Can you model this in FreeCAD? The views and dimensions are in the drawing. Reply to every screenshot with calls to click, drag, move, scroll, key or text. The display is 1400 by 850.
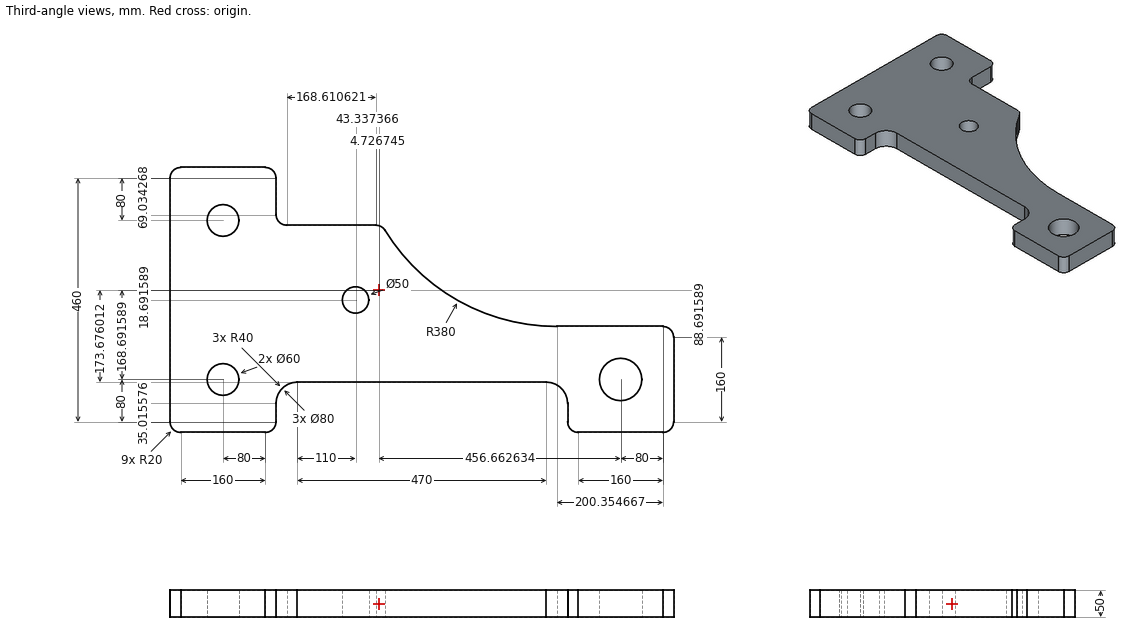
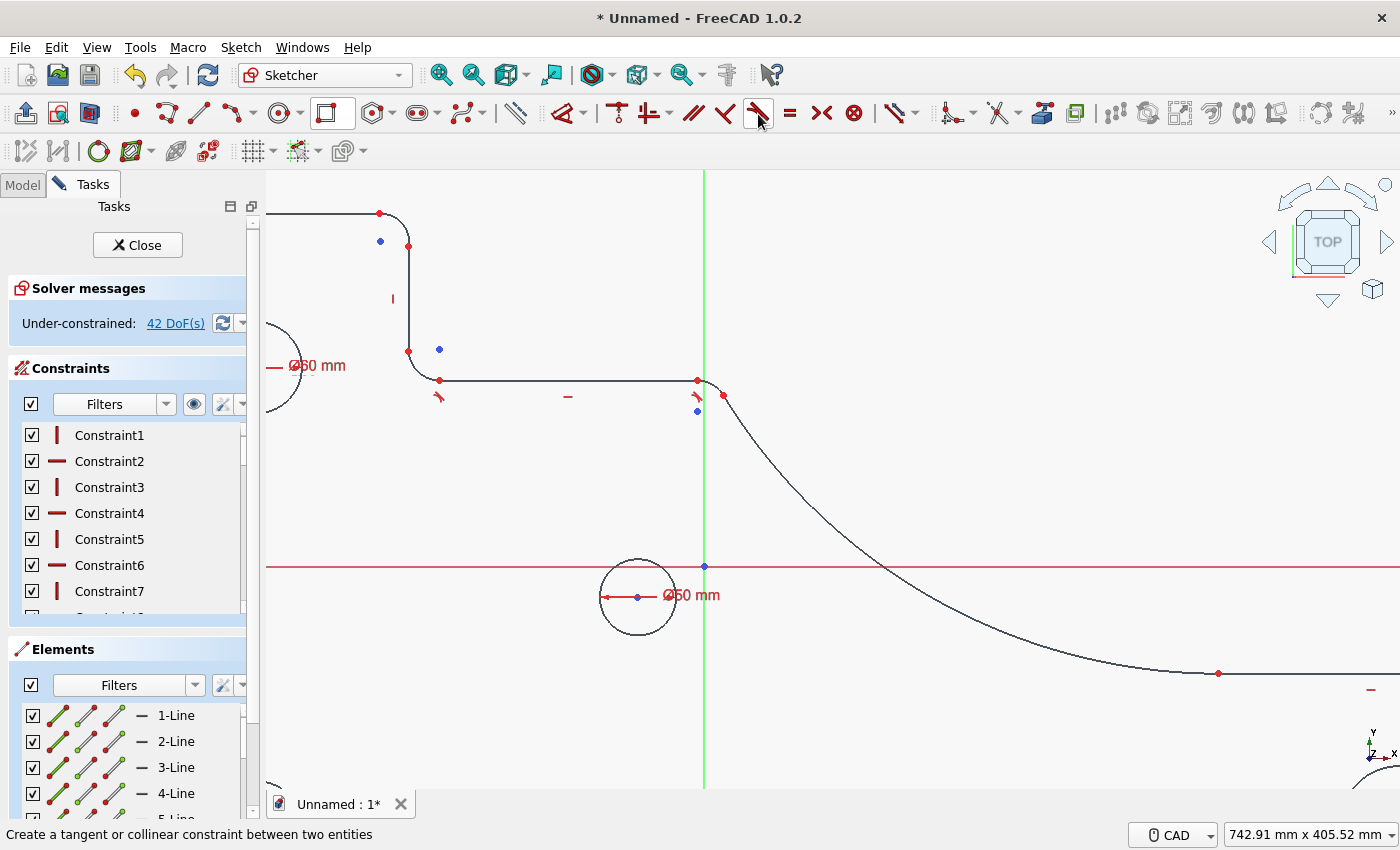
click(409, 320)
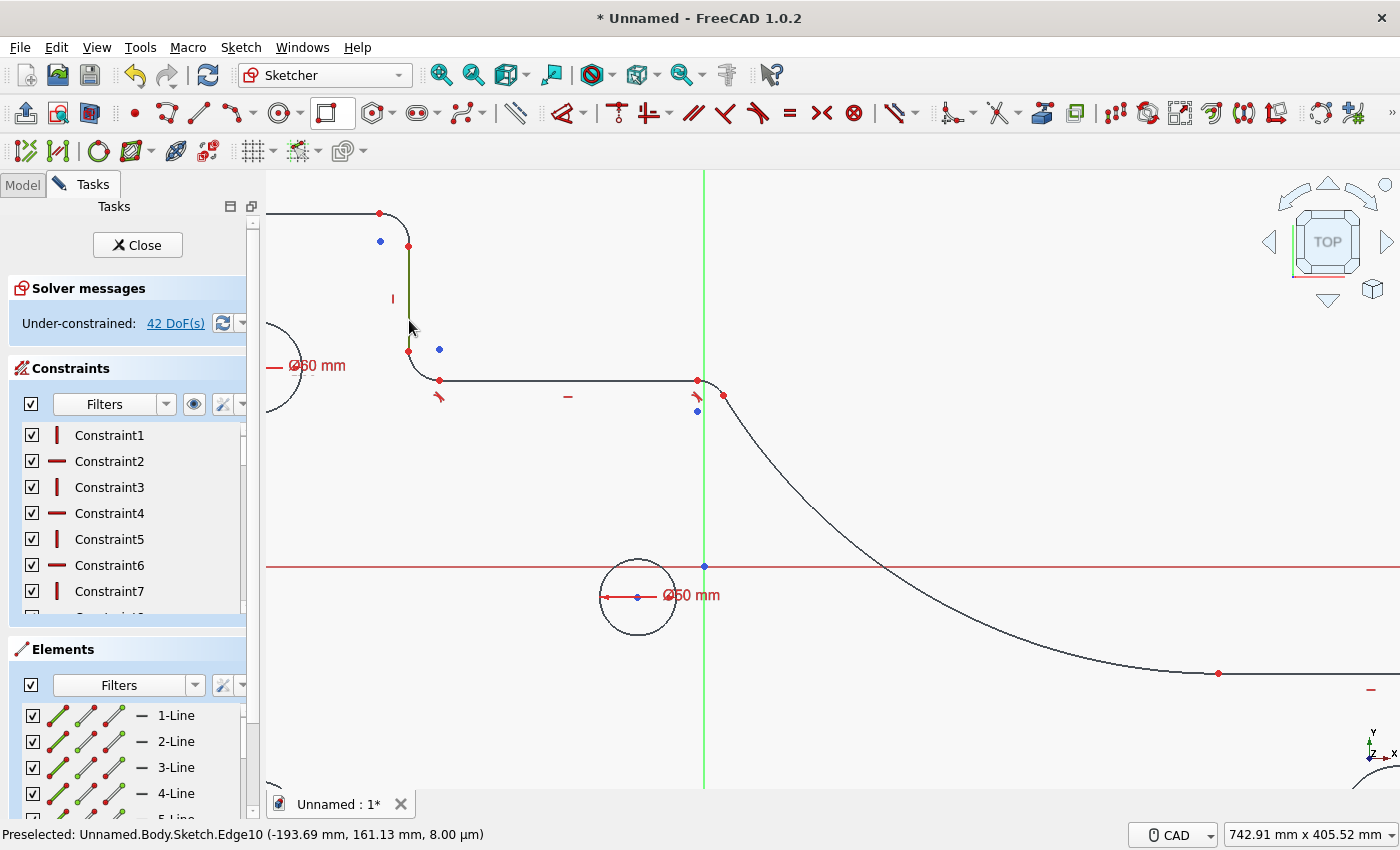
click(413, 365)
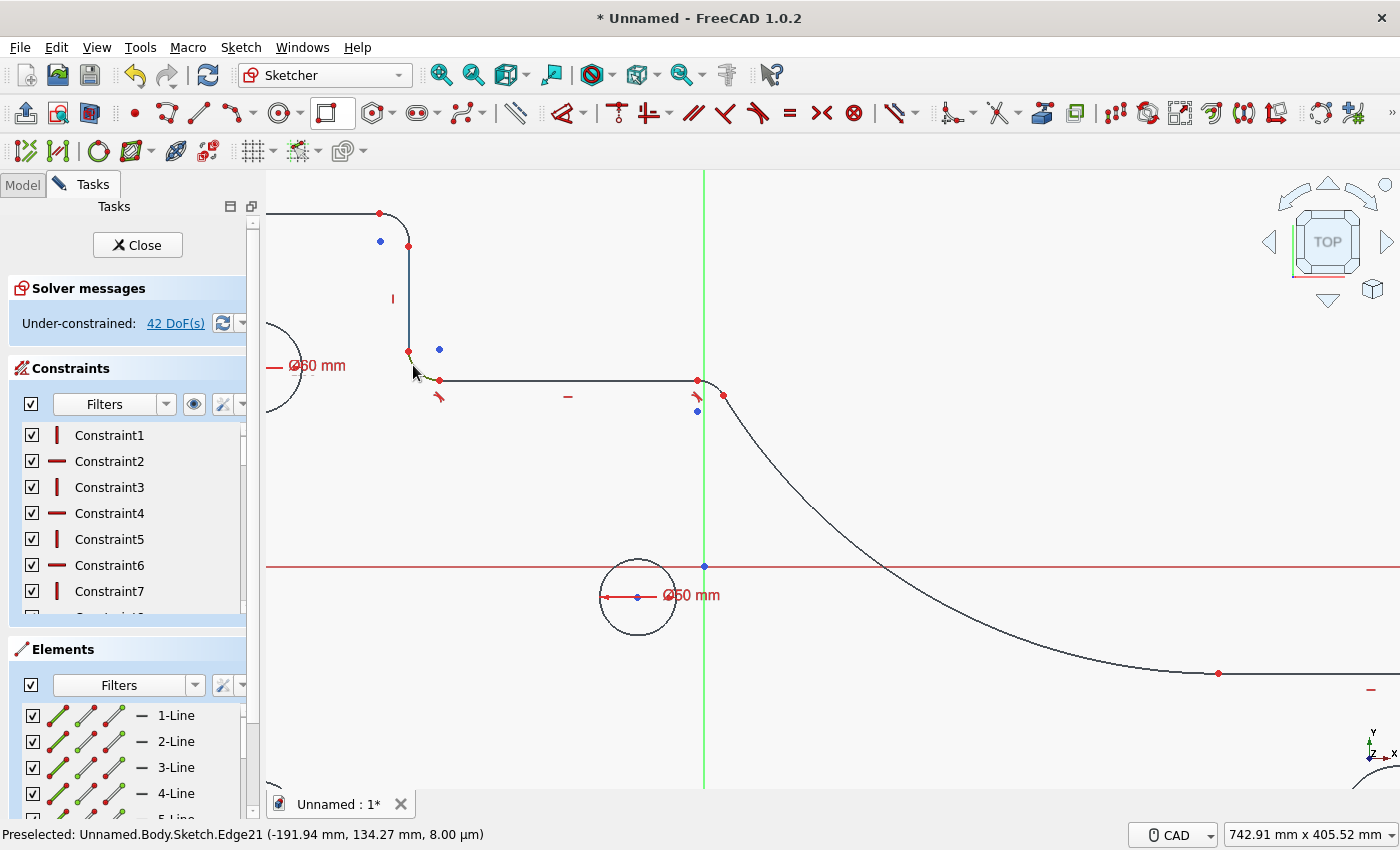
click(758, 114)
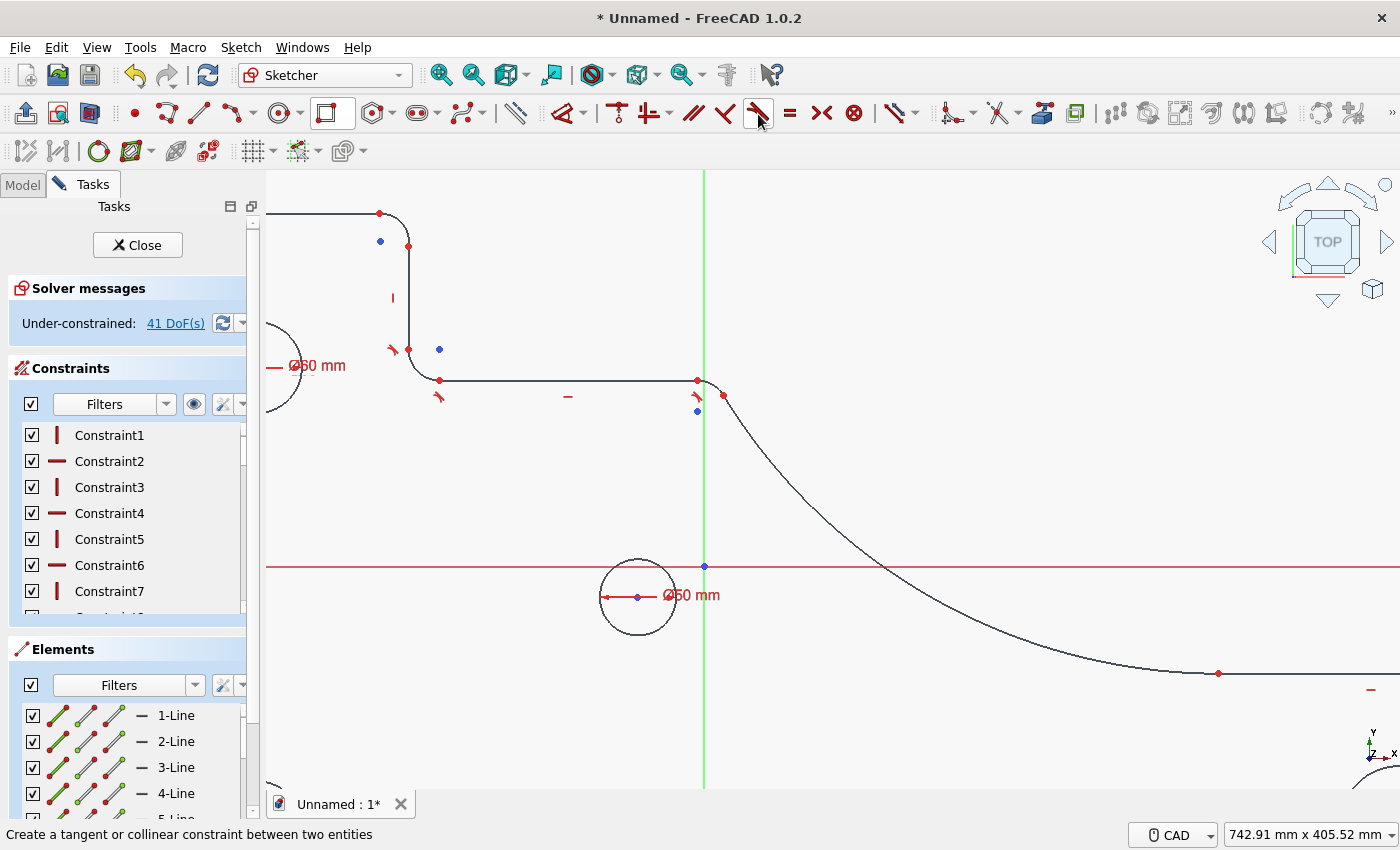
click(409, 318)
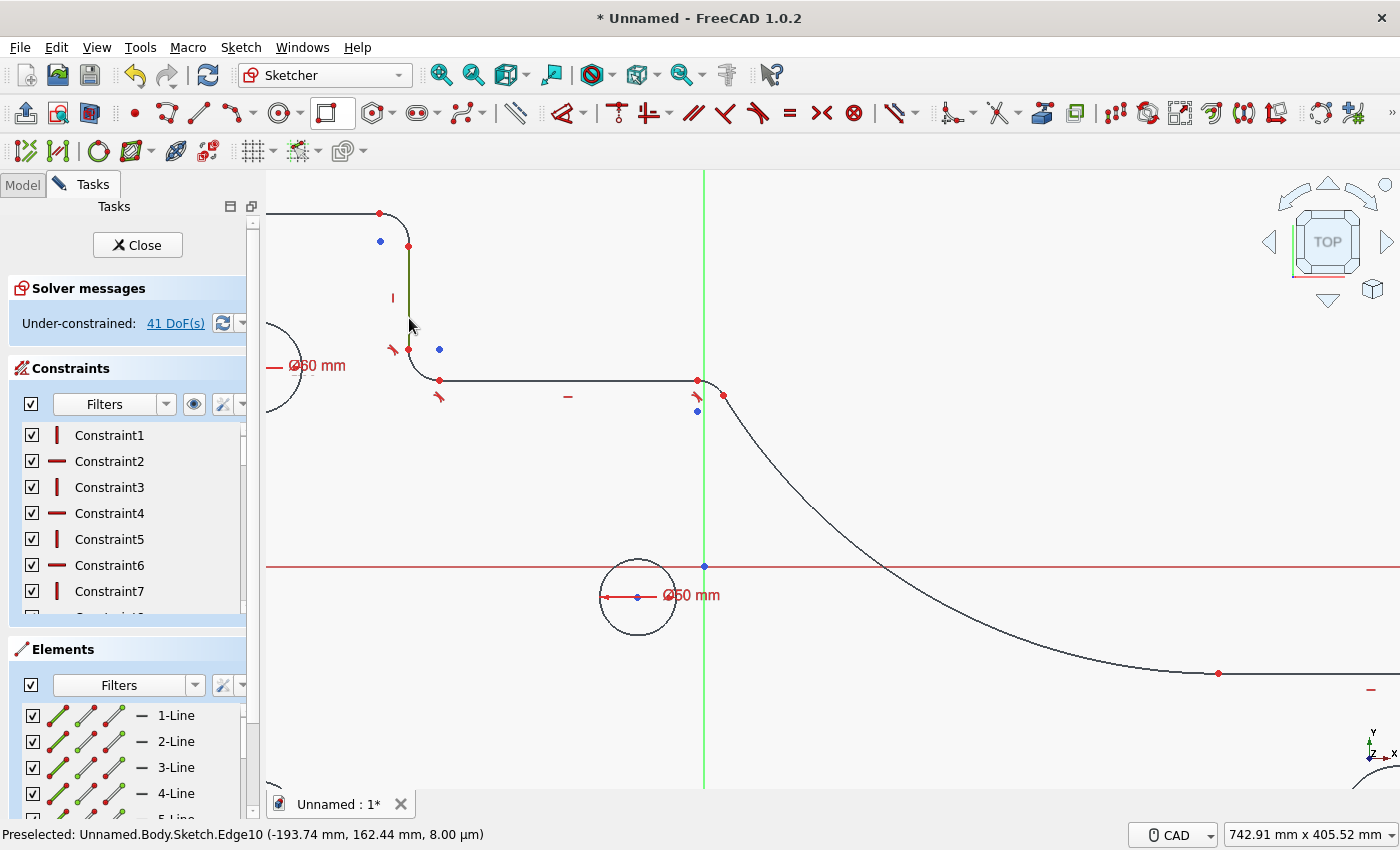
click(407, 232)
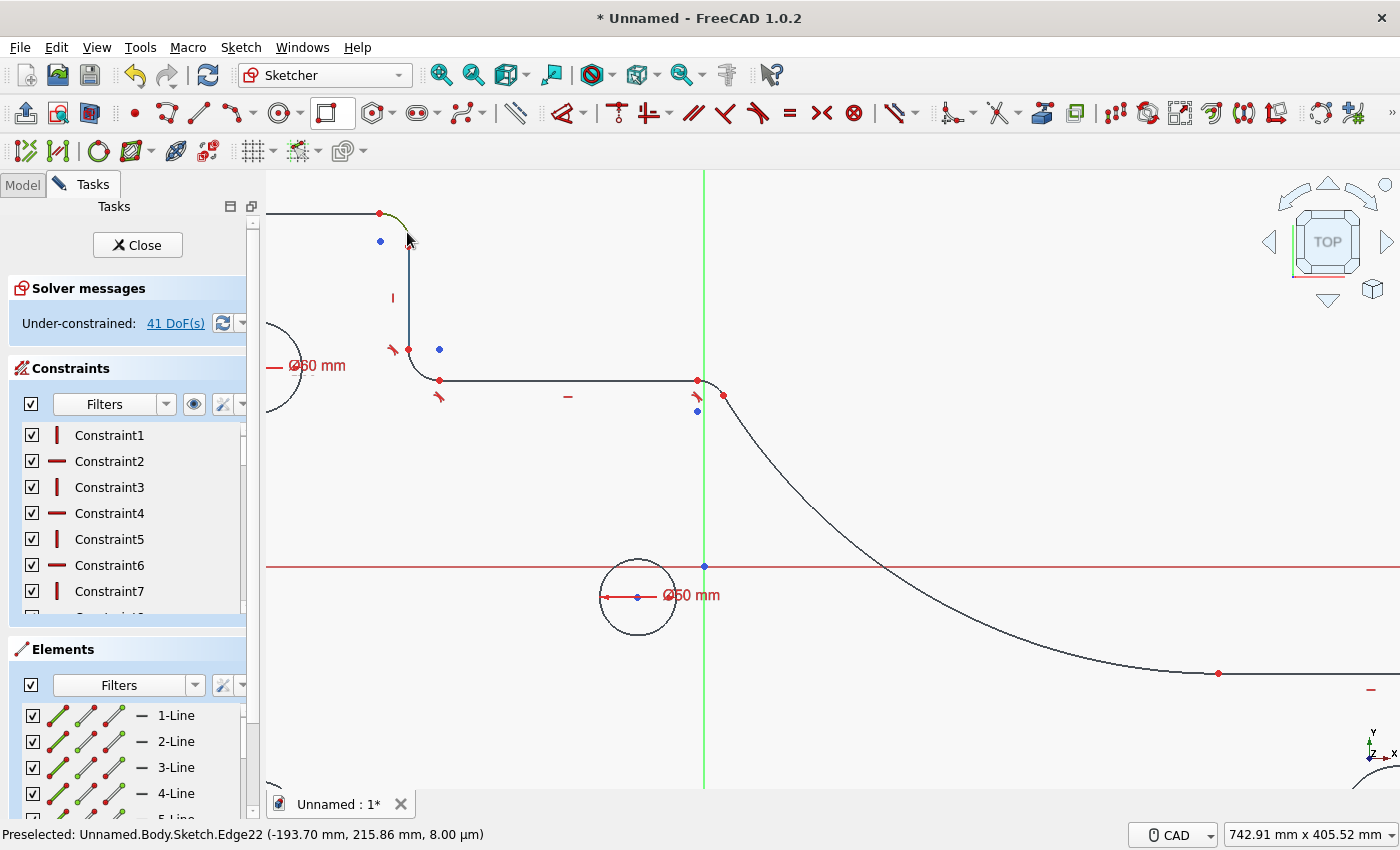
click(758, 114)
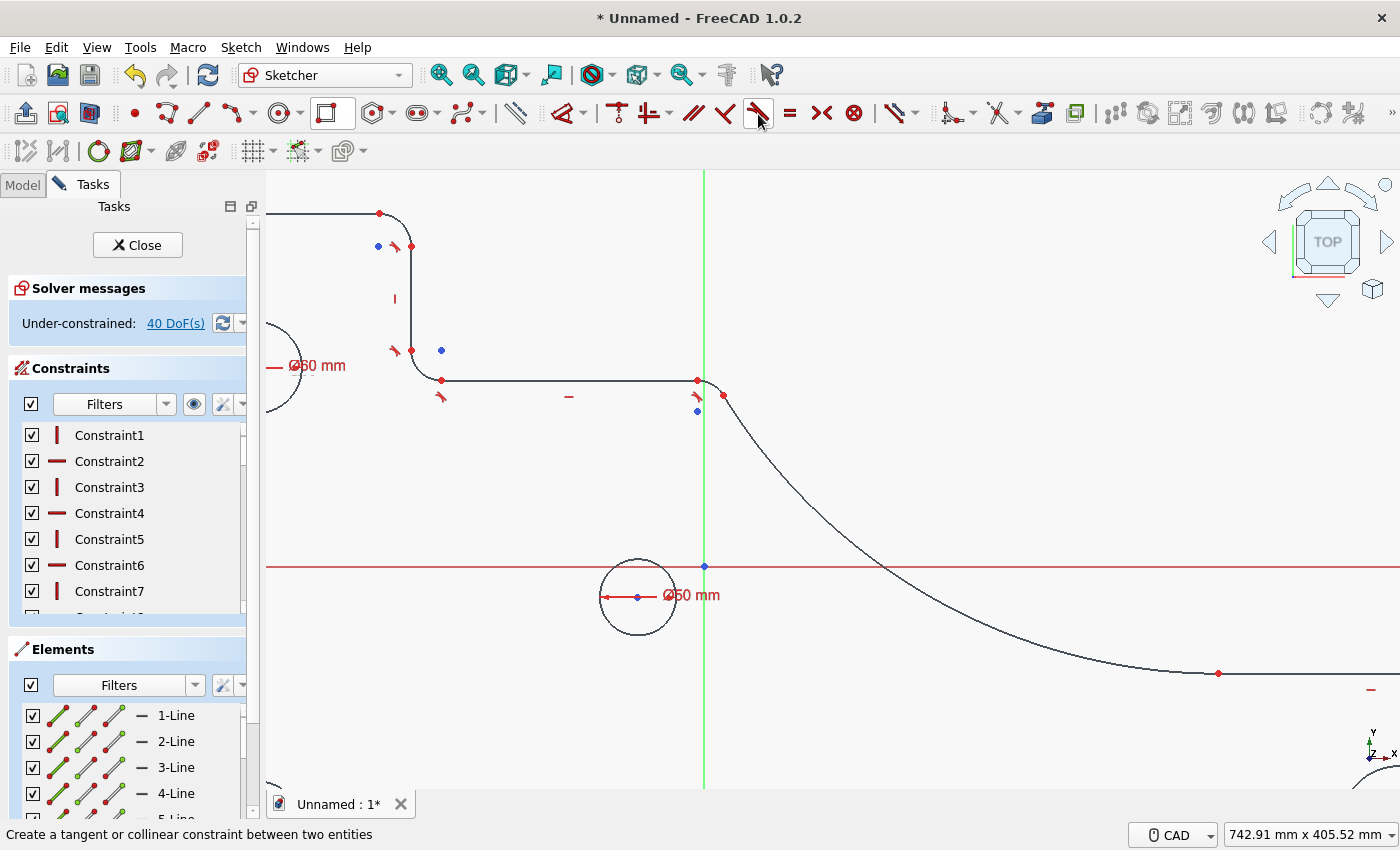
click(306, 214)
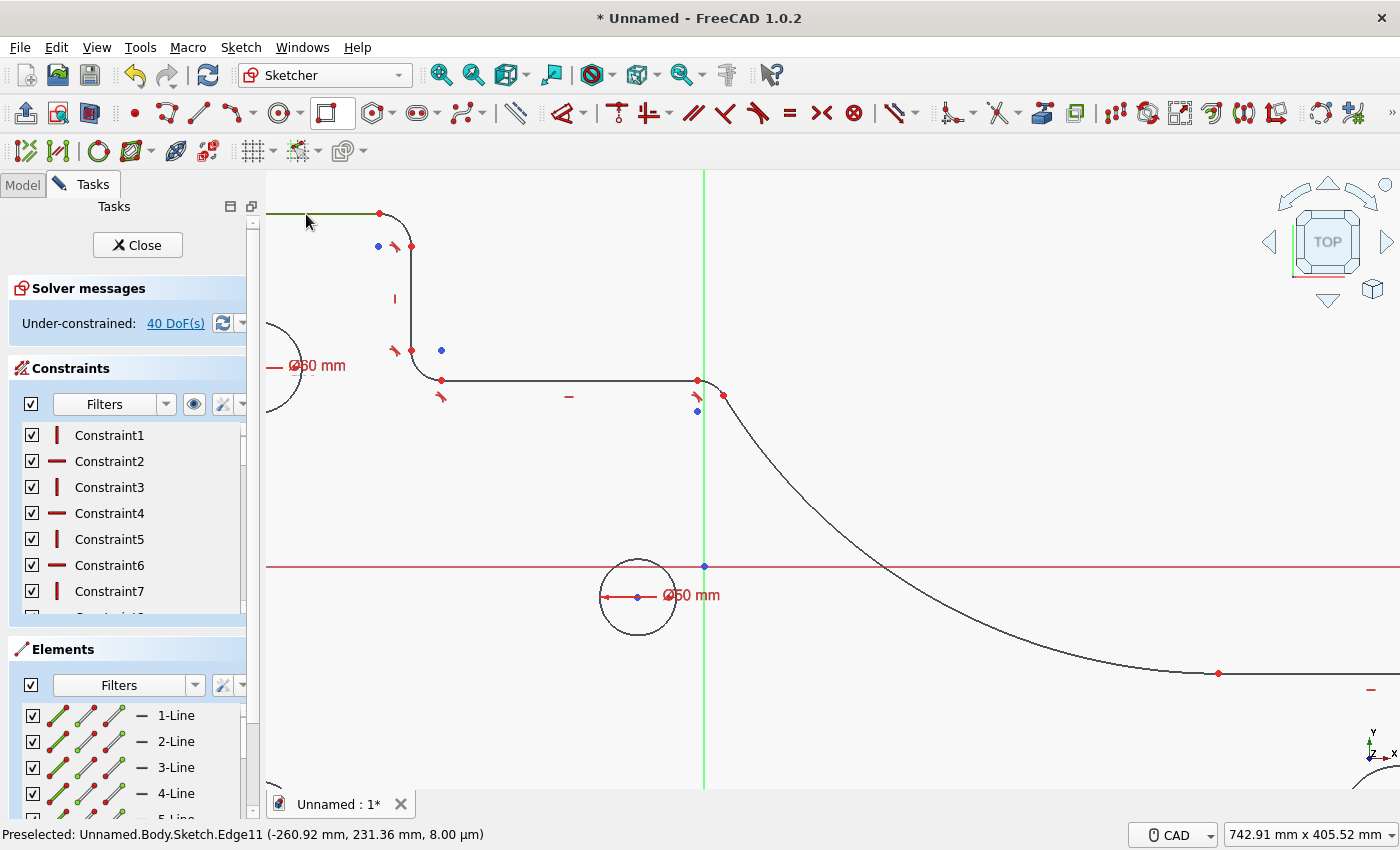
click(408, 232)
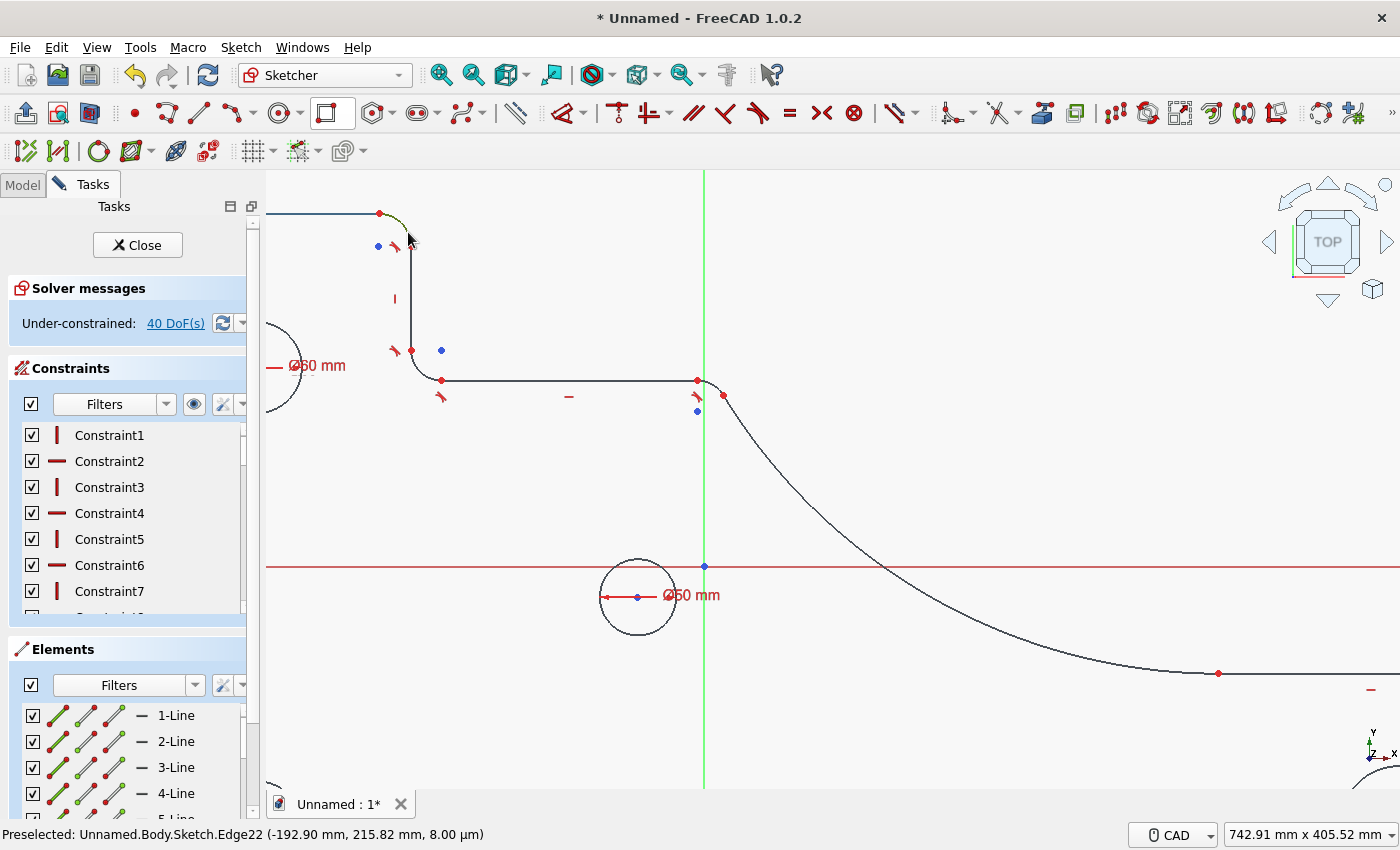
click(758, 114)